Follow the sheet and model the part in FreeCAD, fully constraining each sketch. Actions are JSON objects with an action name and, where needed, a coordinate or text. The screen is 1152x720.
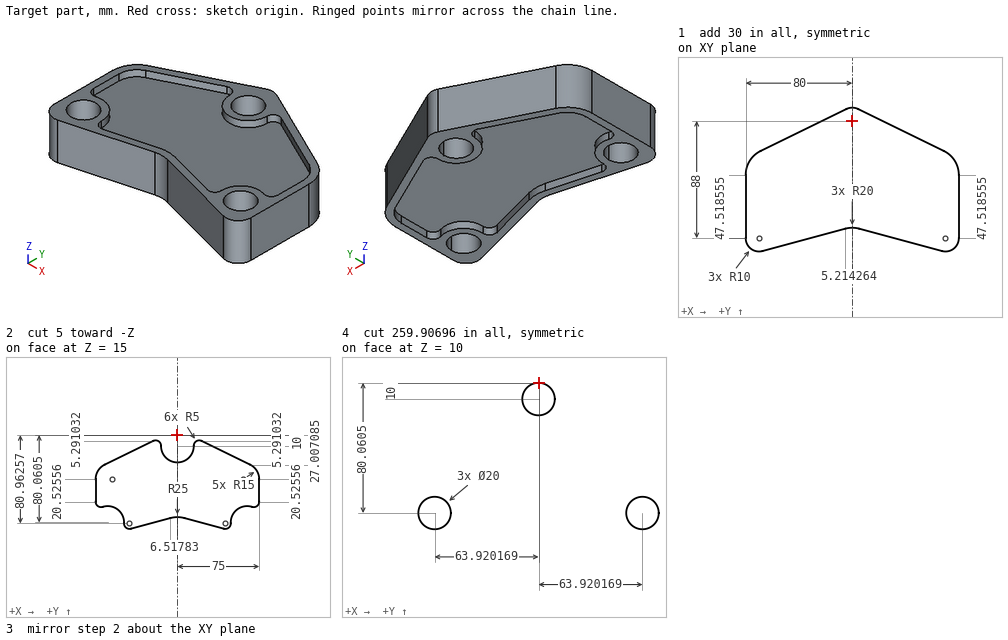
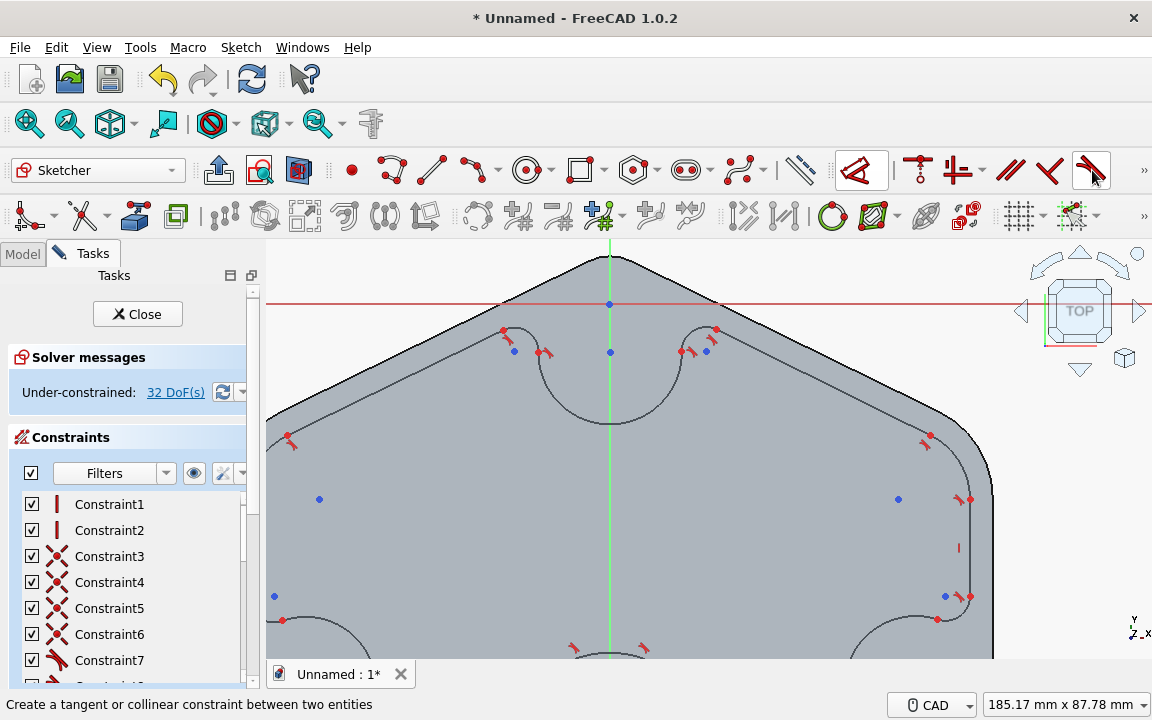
{"action": "scroll", "coordinate": [703, 326], "scroll_direction": "down", "scroll_amount": 2}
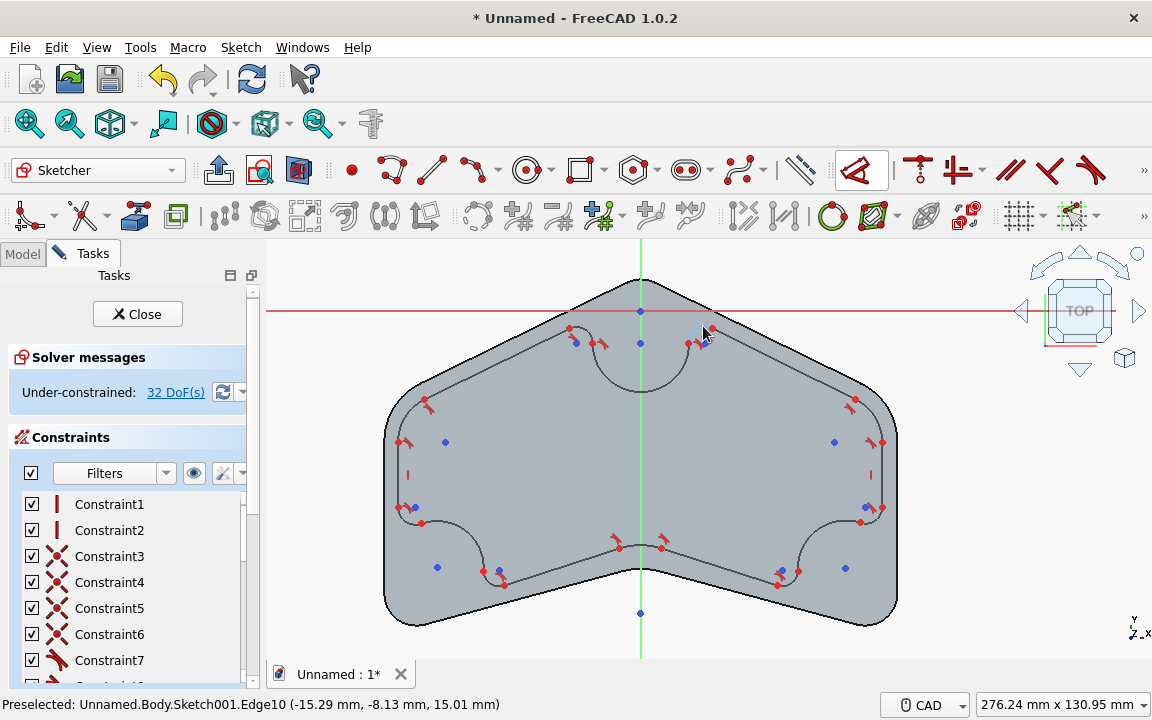
{"action": "scroll", "coordinate": [401, 517], "scroll_direction": "up", "scroll_amount": 2}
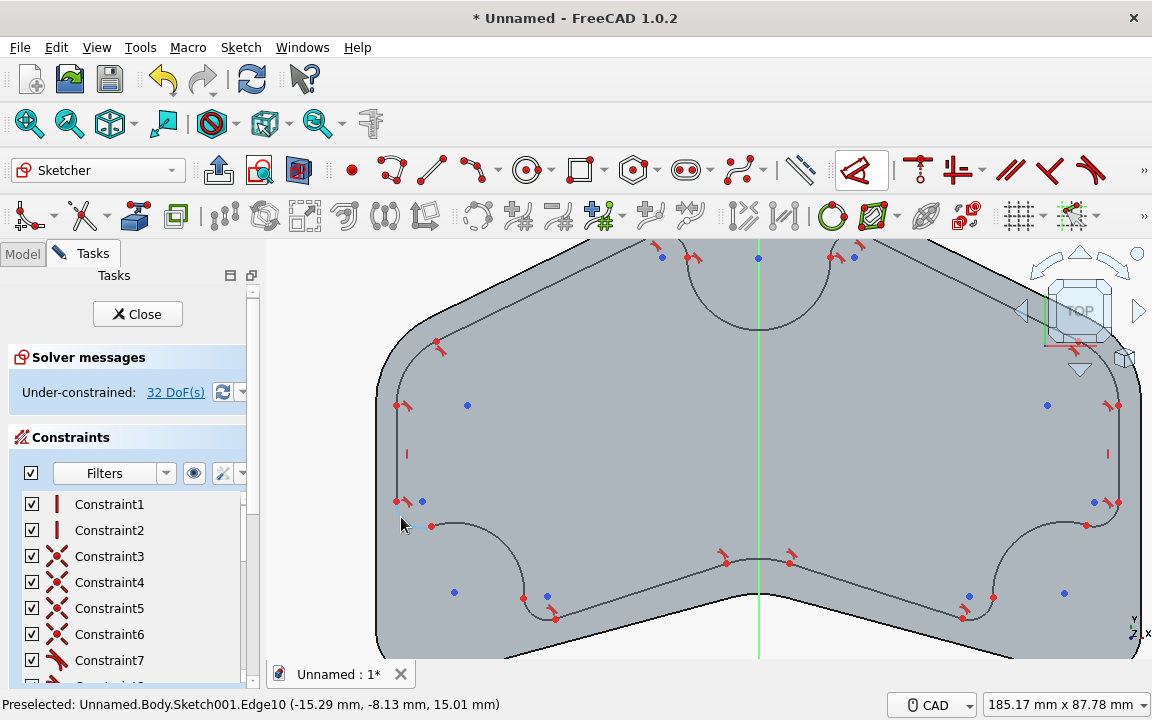
{"action": "left_click", "coordinate": [401, 516]}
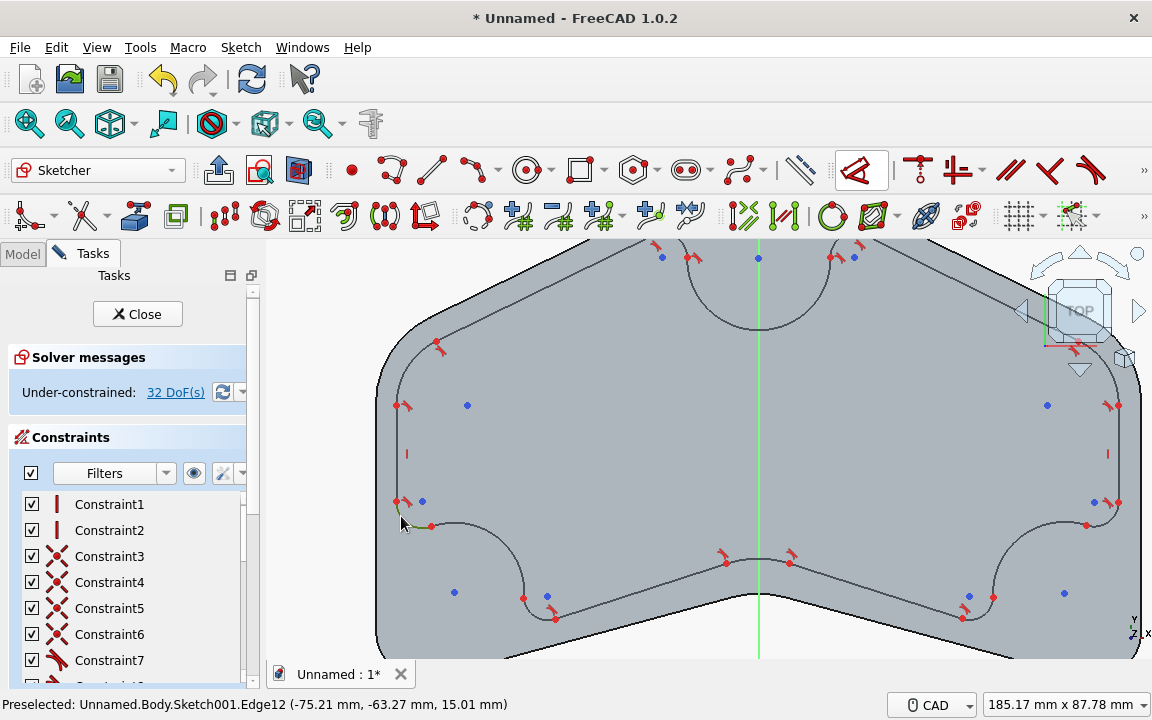
{"action": "left_click", "coordinate": [515, 558]}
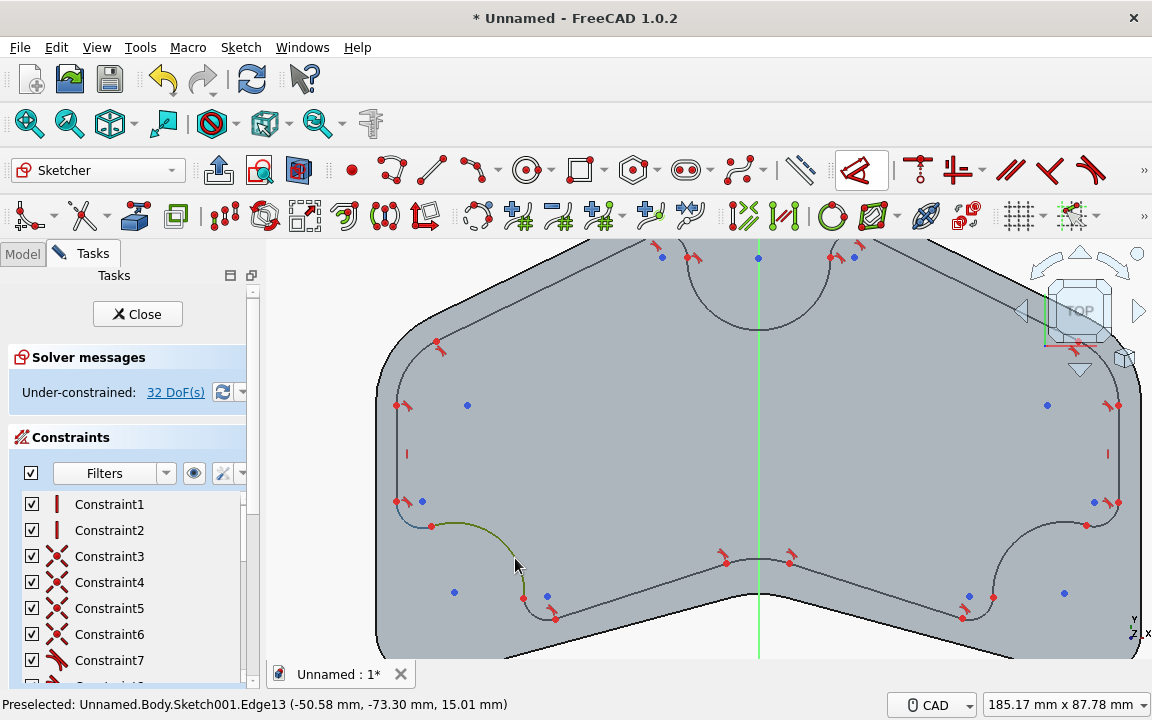
{"action": "left_click", "coordinate": [1092, 170]}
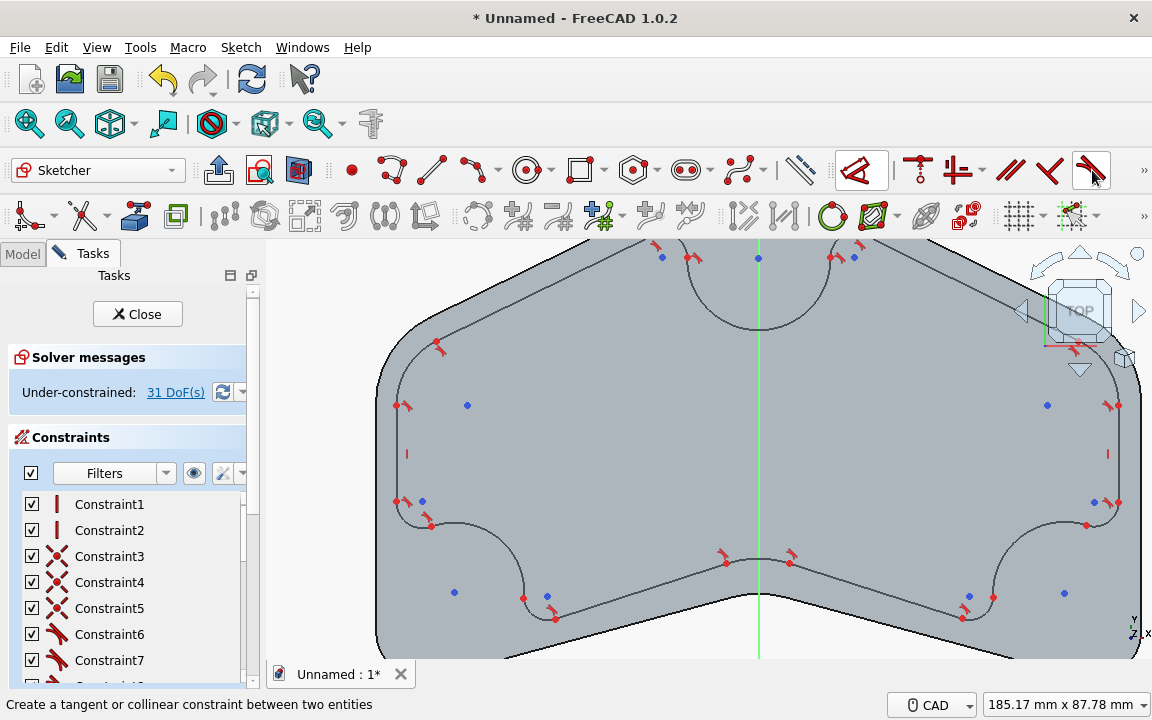
{"action": "left_click", "coordinate": [515, 558]}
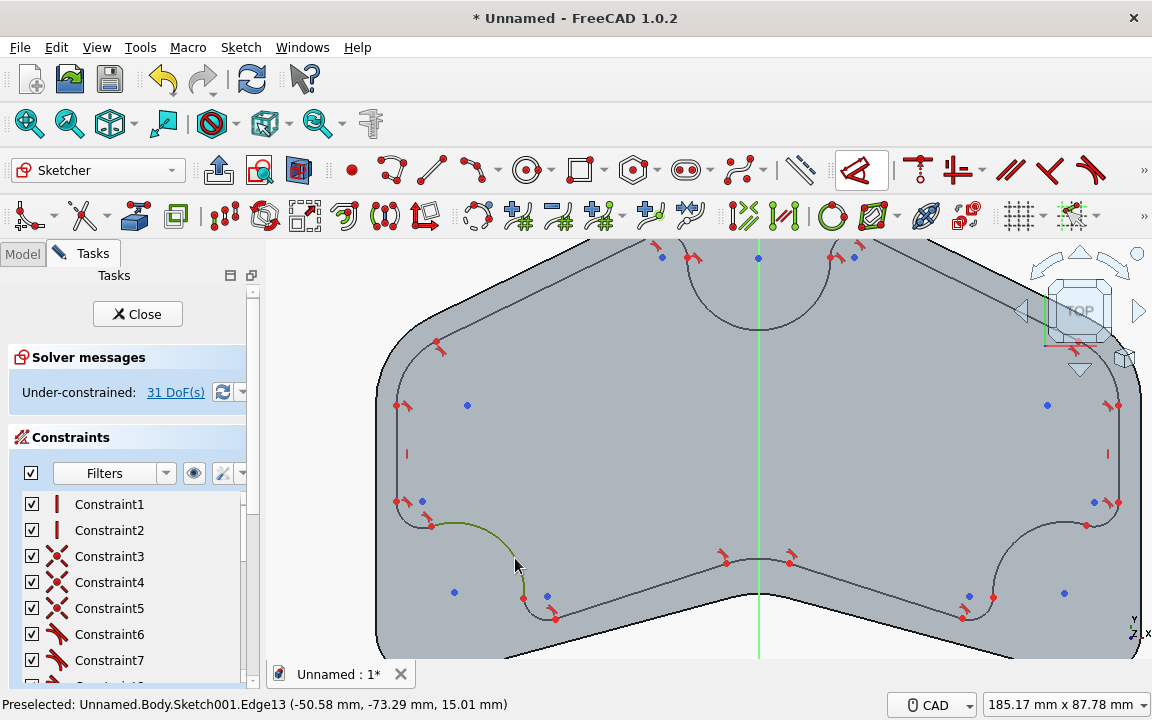
{"action": "left_click", "coordinate": [528, 610]}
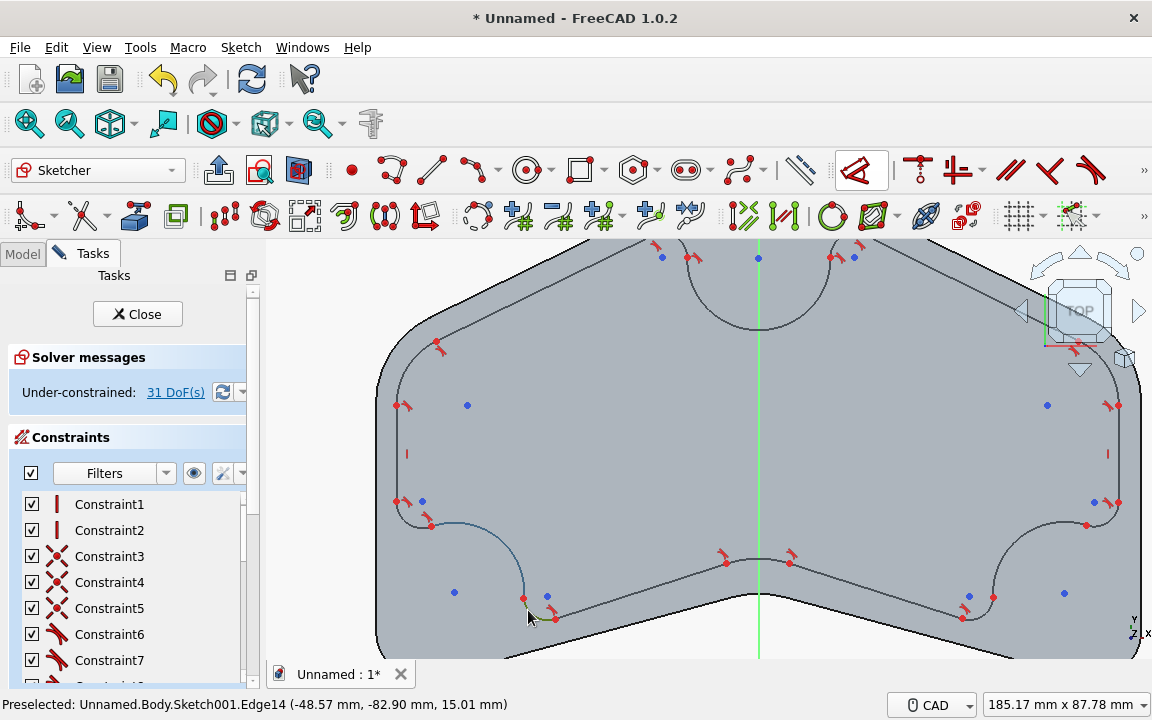
{"action": "left_click", "coordinate": [1092, 170]}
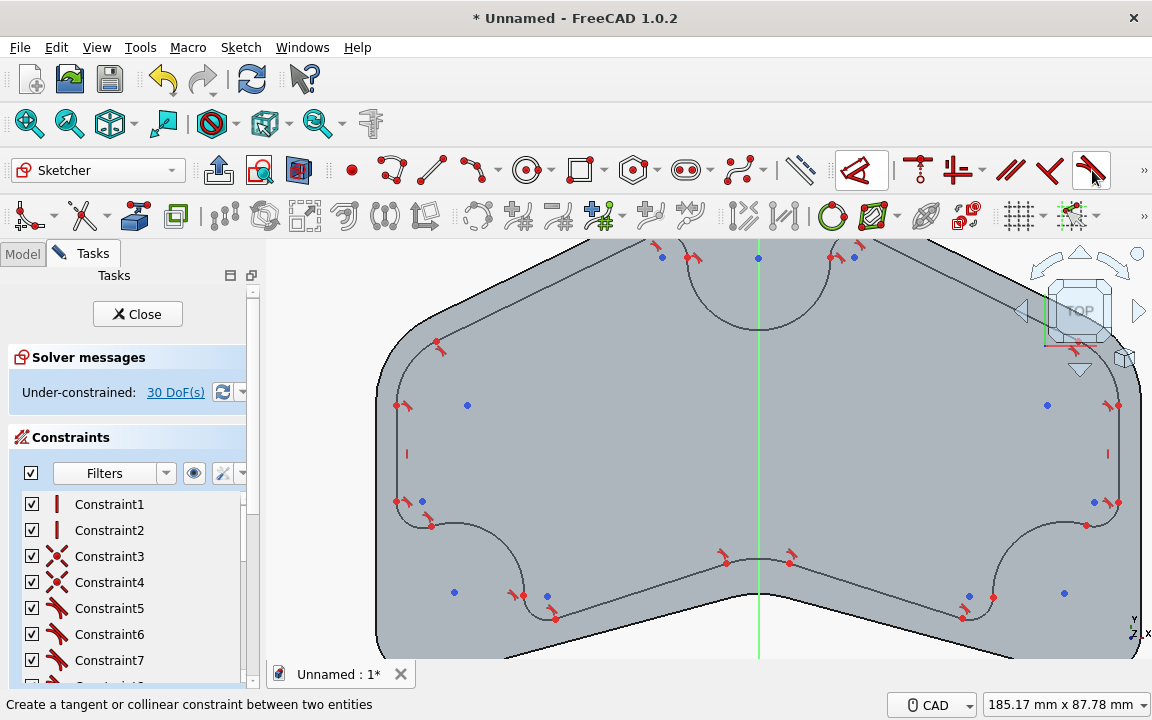
{"action": "left_click", "coordinate": [975, 619]}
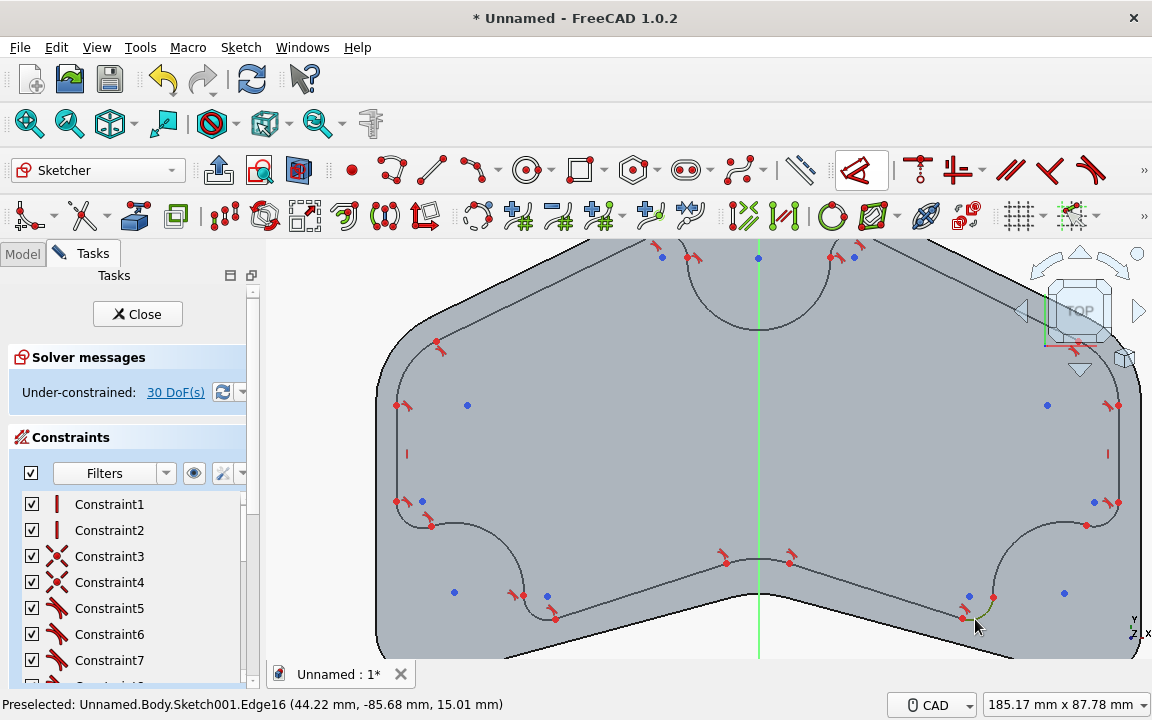
{"action": "scroll", "coordinate": [400, 518], "scroll_direction": "down", "scroll_amount": 2}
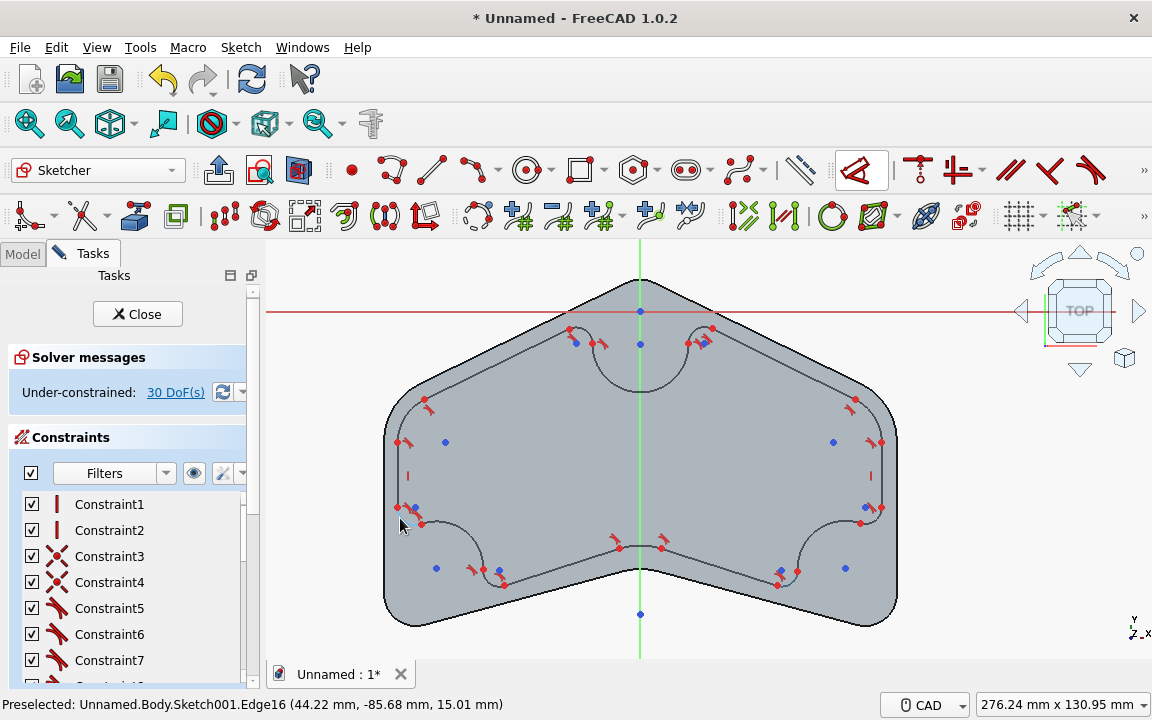
{"action": "left_click", "coordinate": [833, 523]}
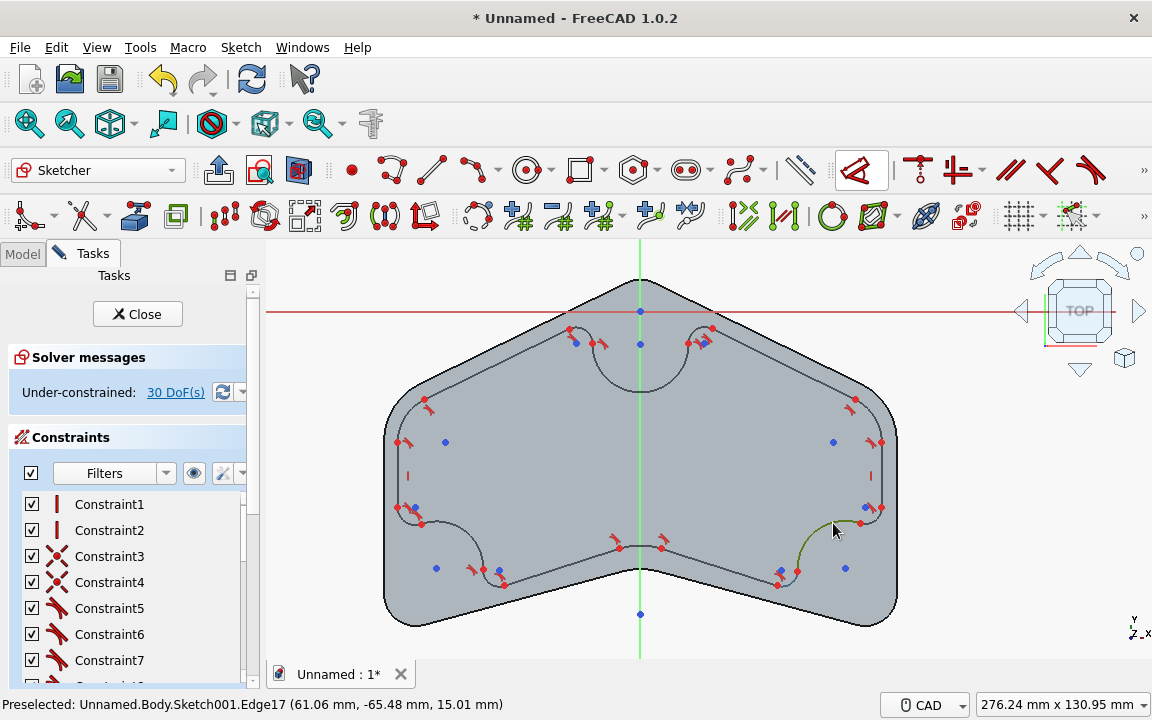
{"action": "key", "text": "t"}